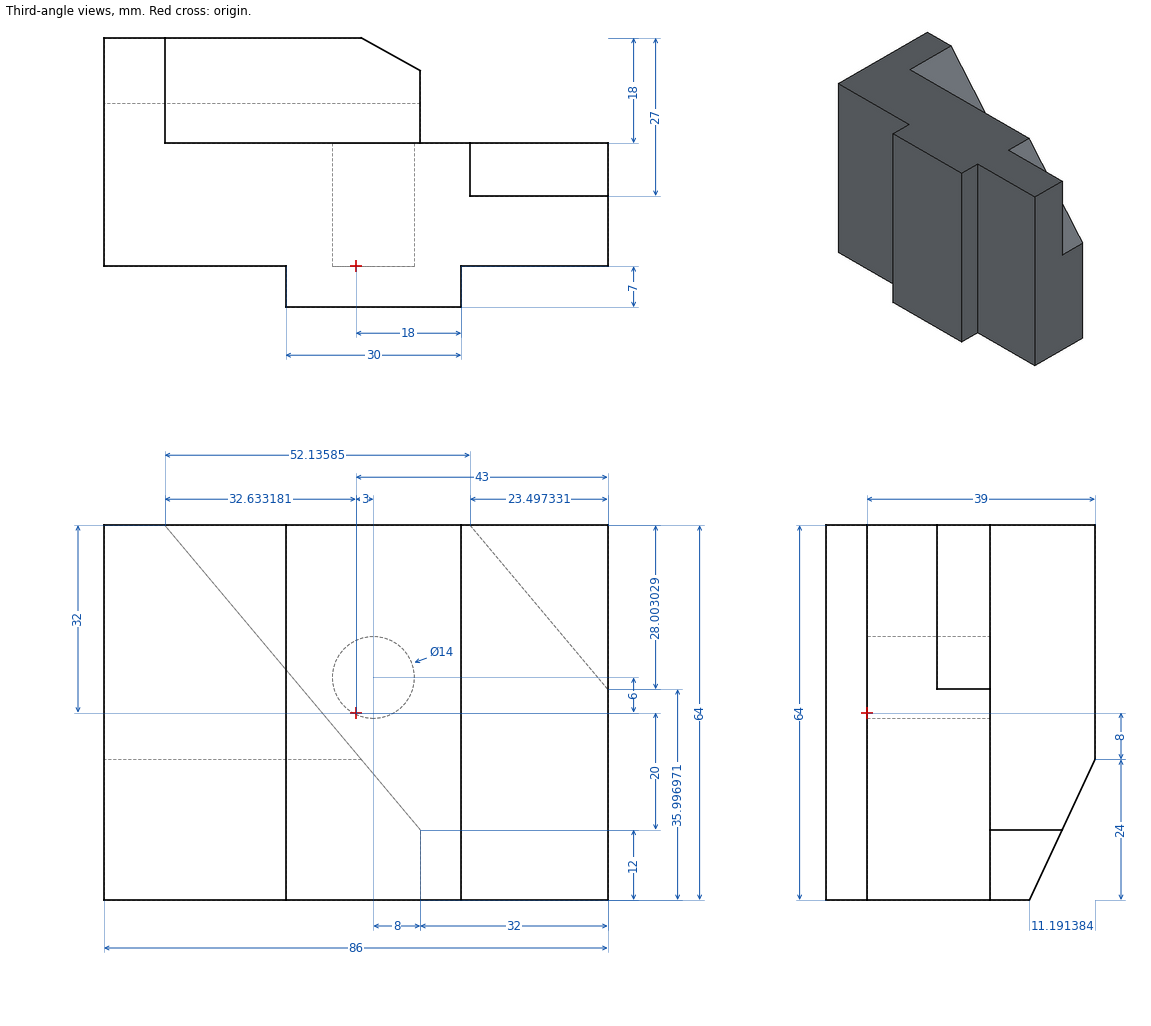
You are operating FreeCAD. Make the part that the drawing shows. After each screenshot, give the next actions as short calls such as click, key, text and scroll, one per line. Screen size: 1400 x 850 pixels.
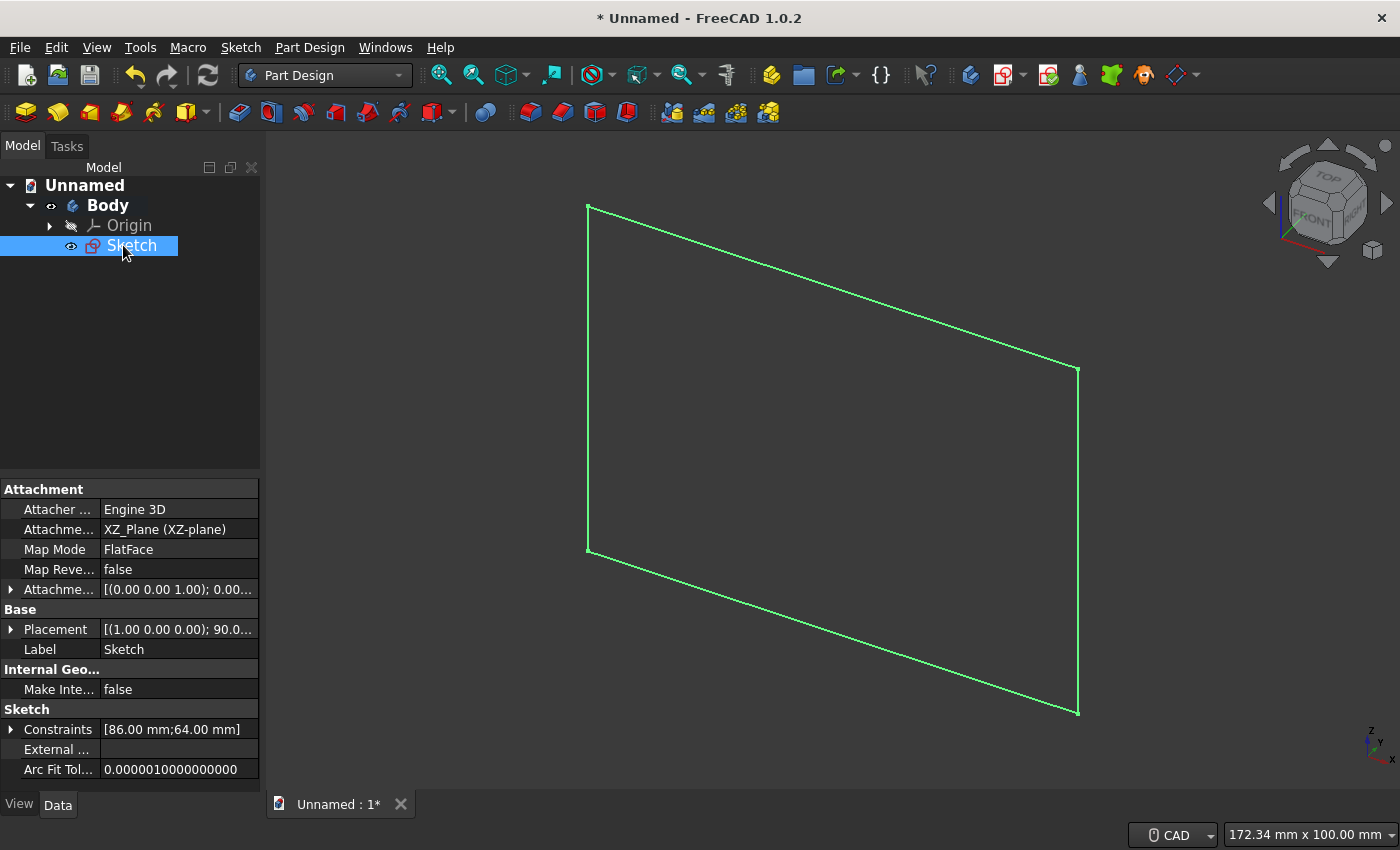
click(26, 112)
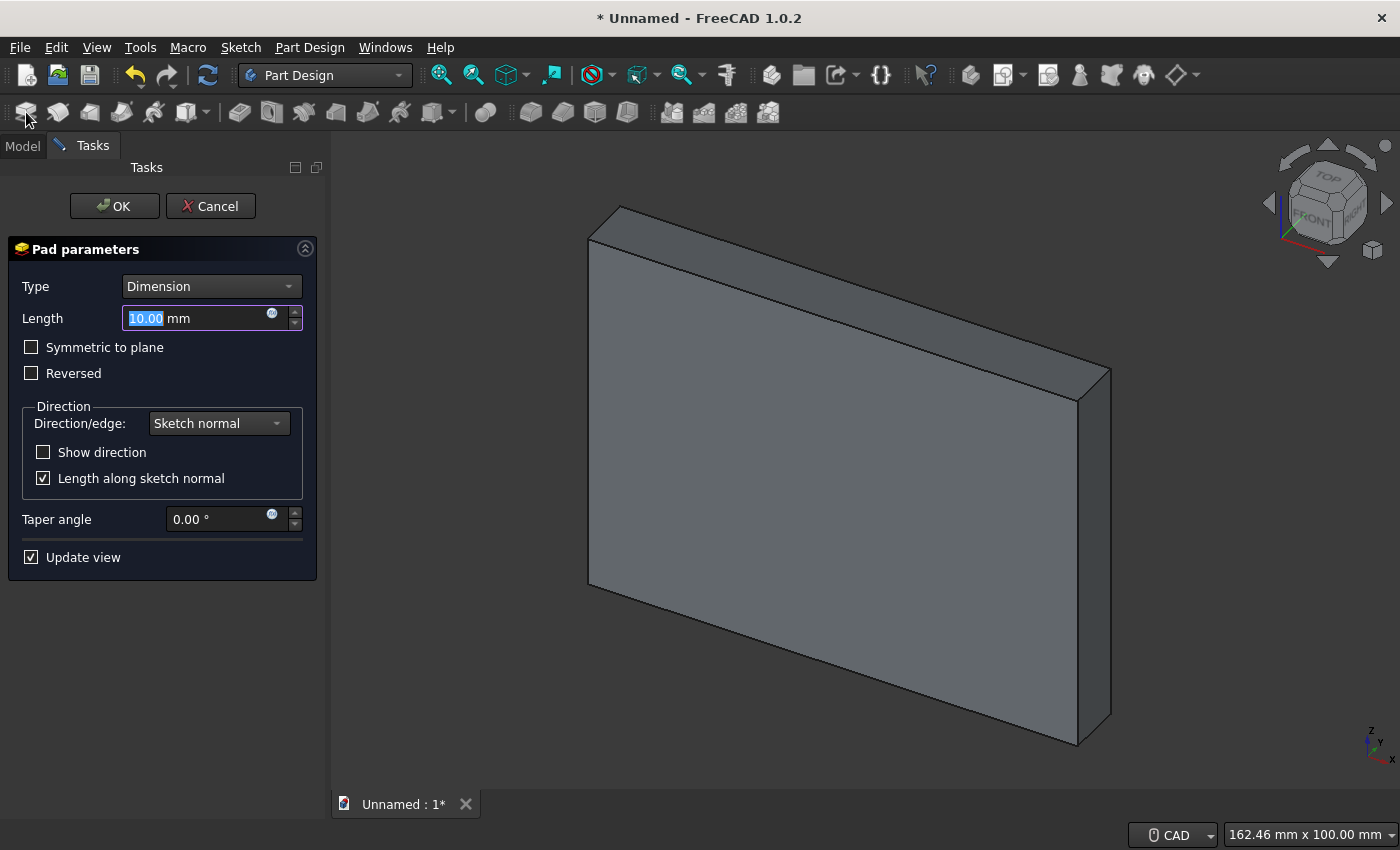
text(39)
key(Tab)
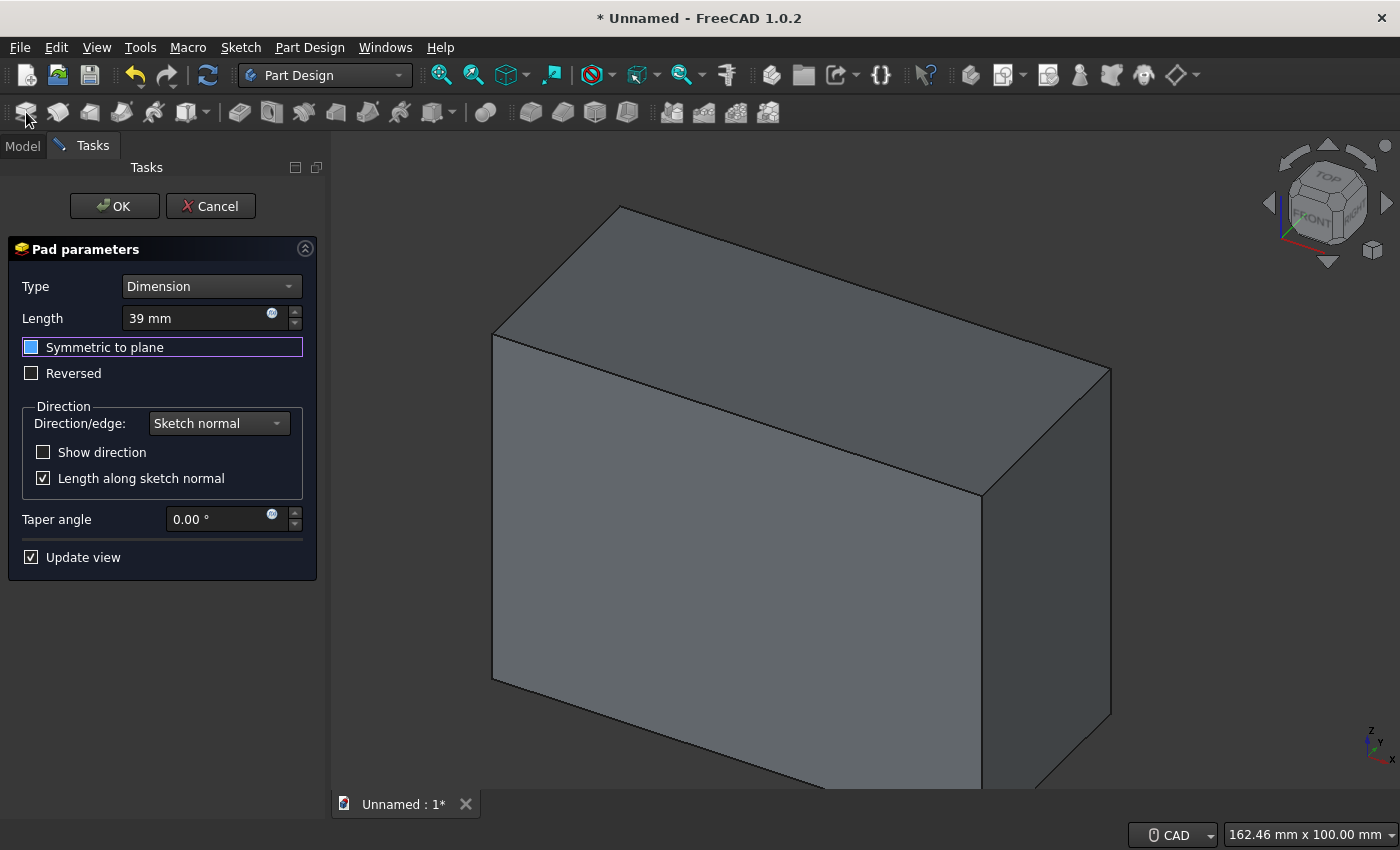
click(30, 373)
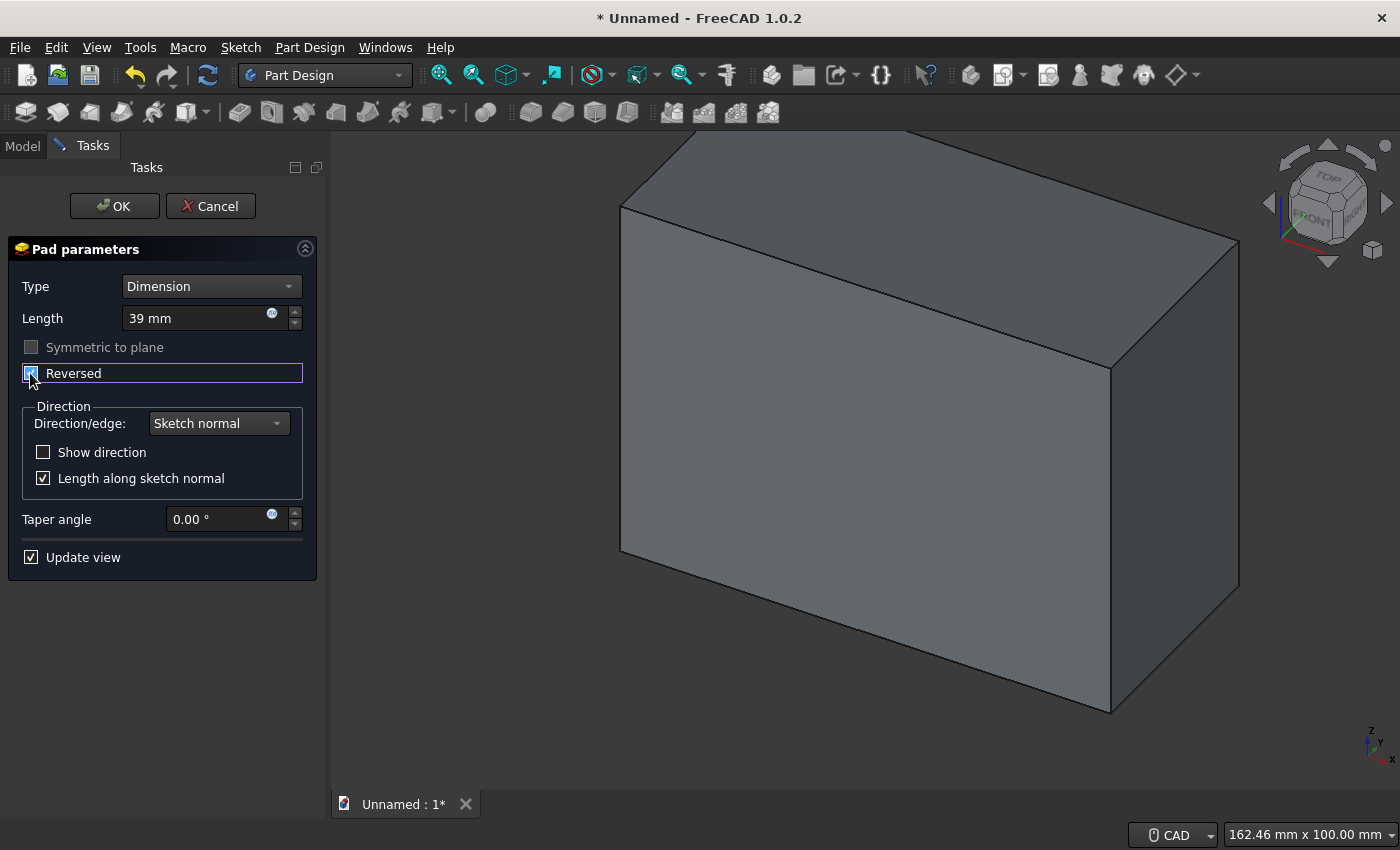
click(115, 206)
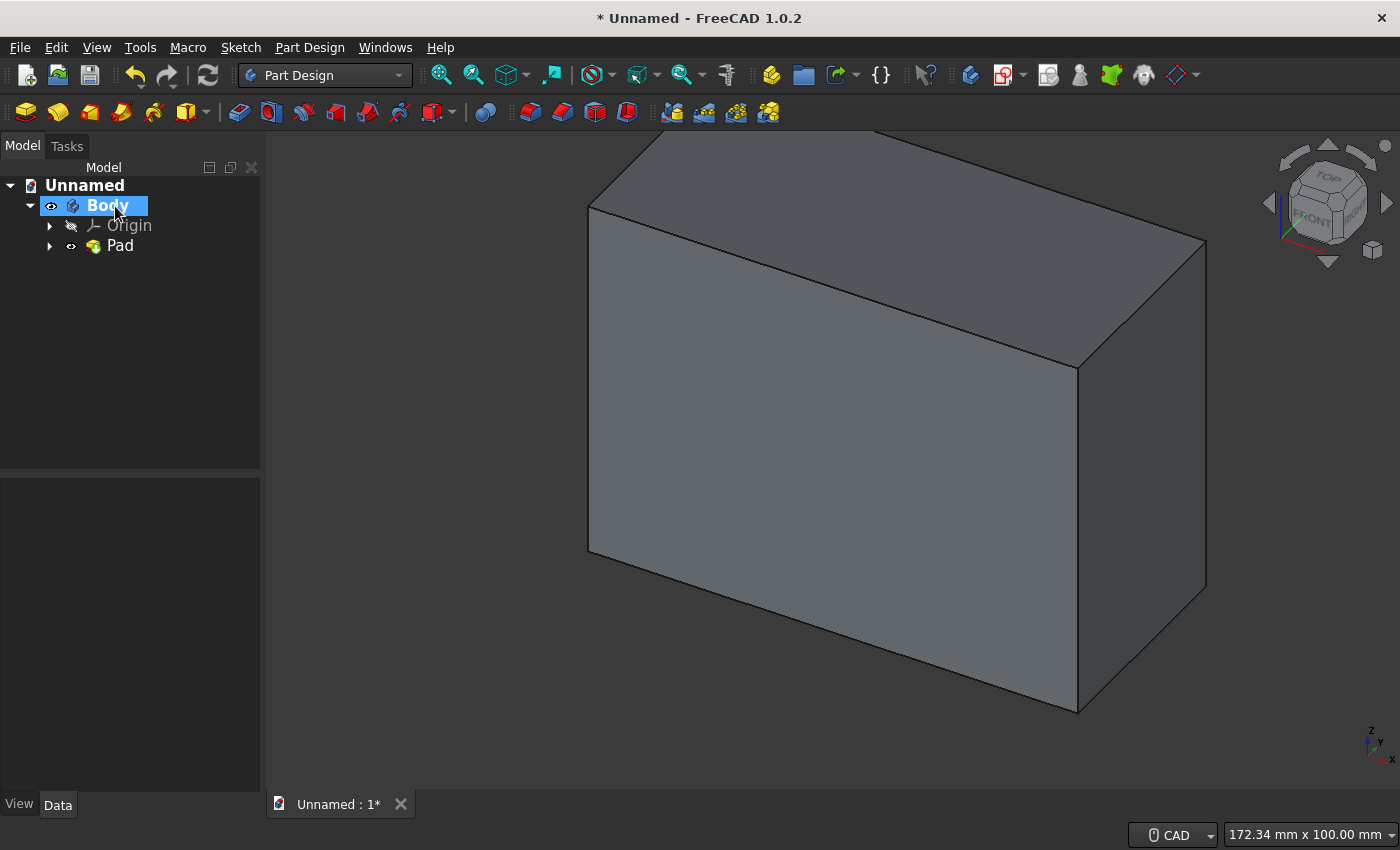
click(442, 76)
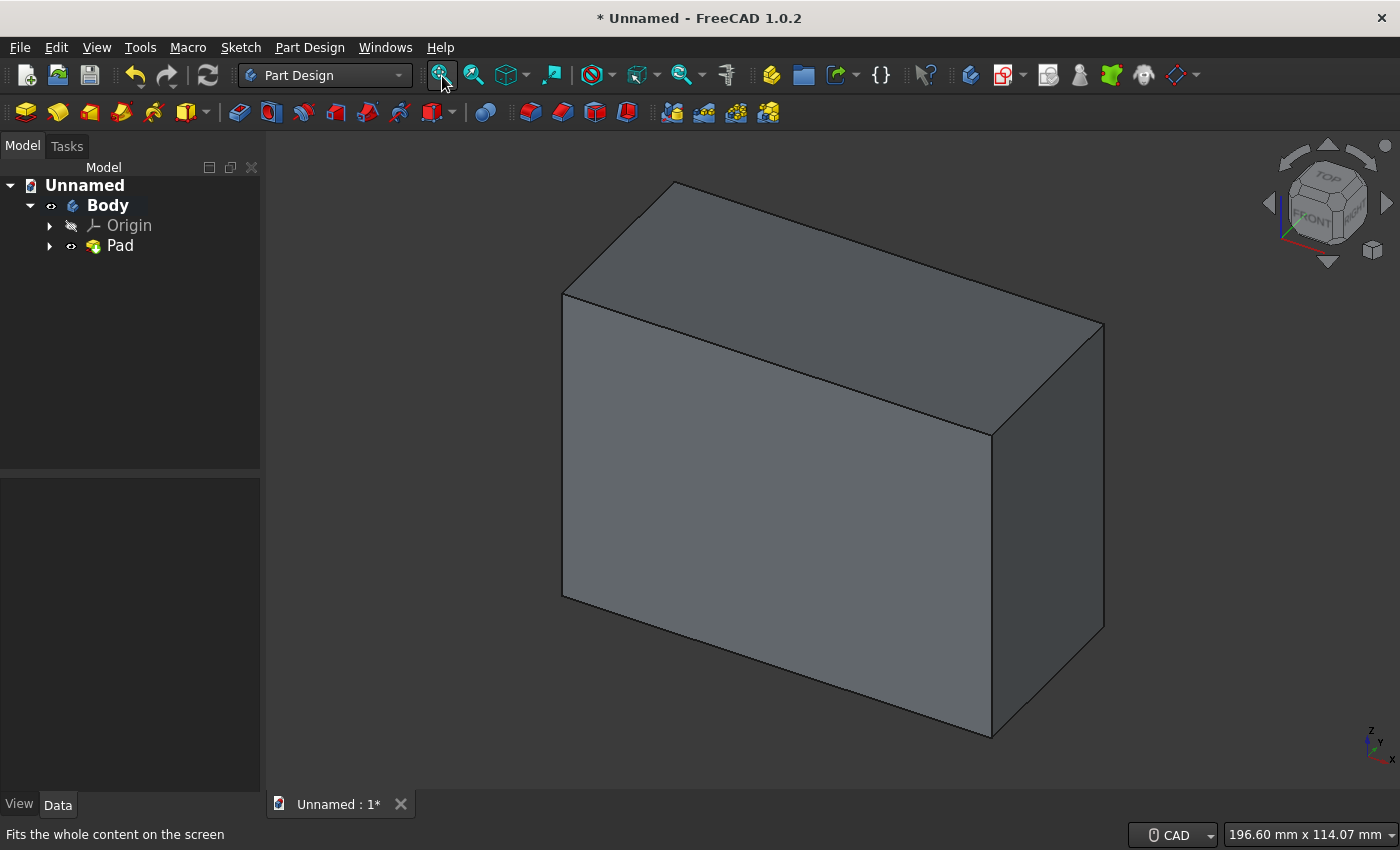
click(1048, 530)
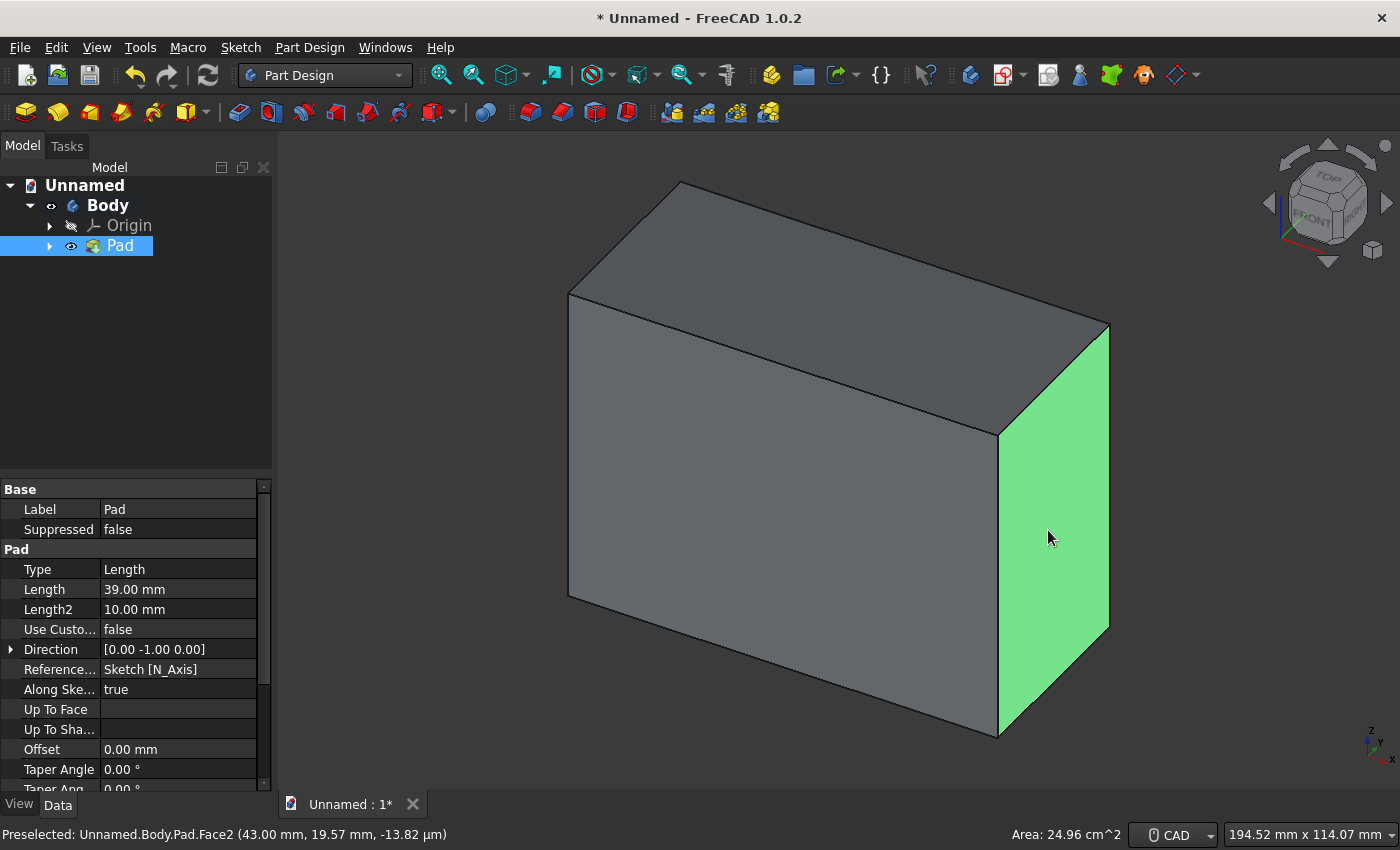
click(1004, 76)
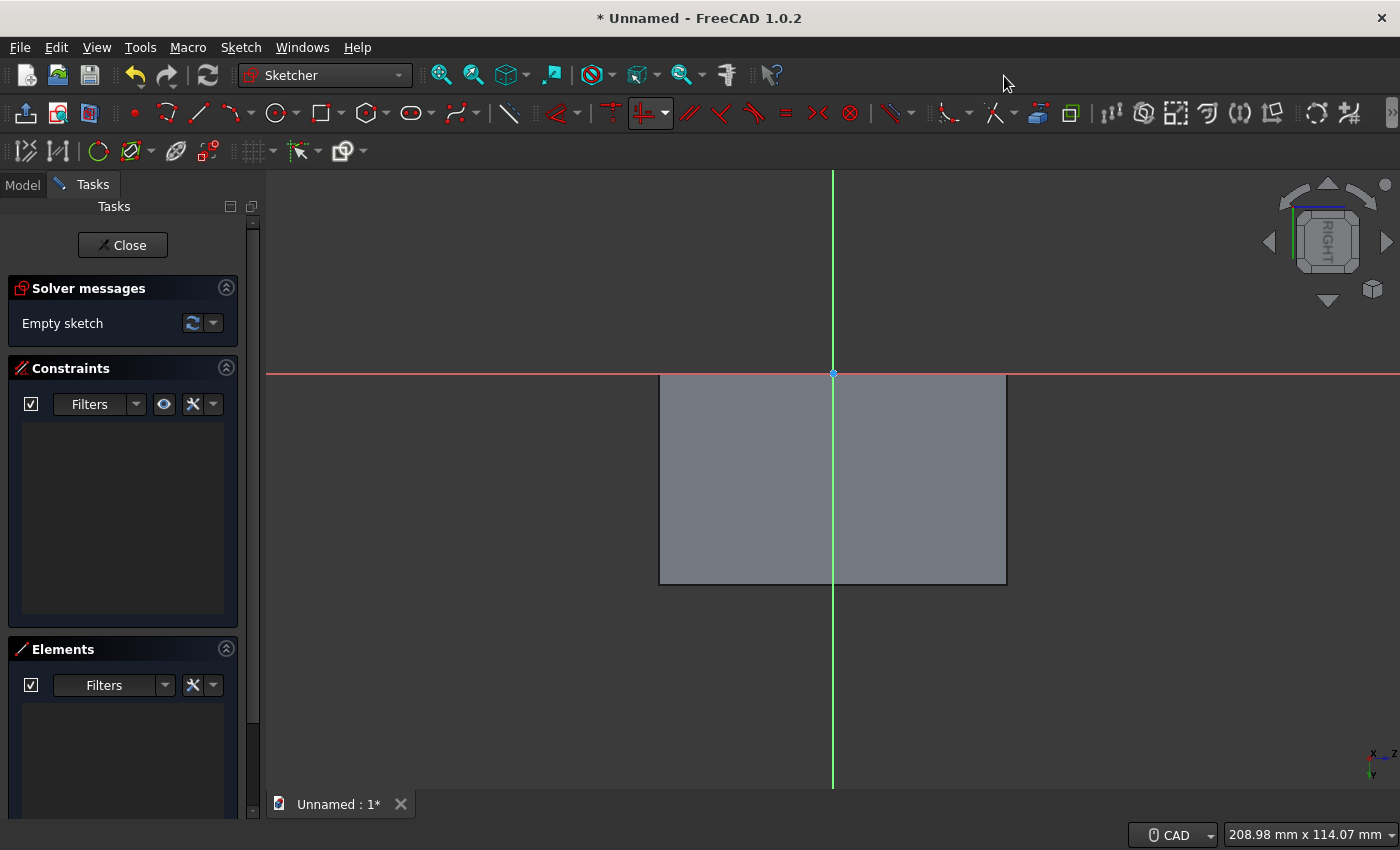
scroll(724, 479, up, 3)